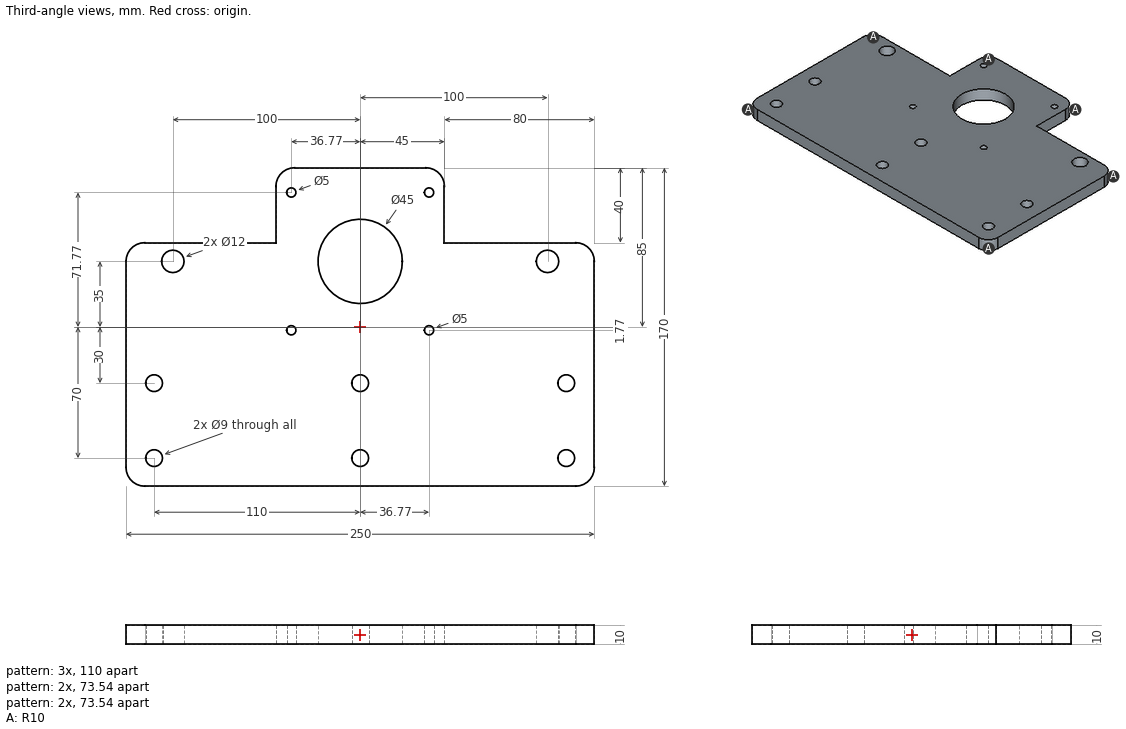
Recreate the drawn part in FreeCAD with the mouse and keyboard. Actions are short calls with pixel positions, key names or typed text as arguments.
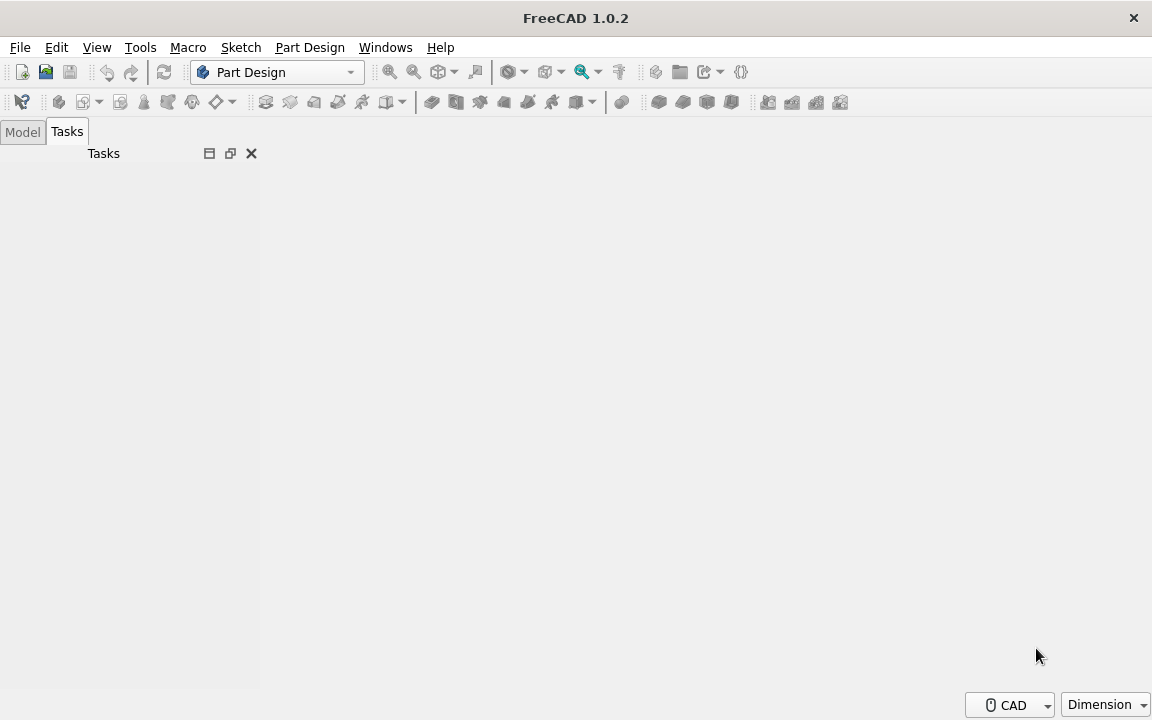
click(22, 72)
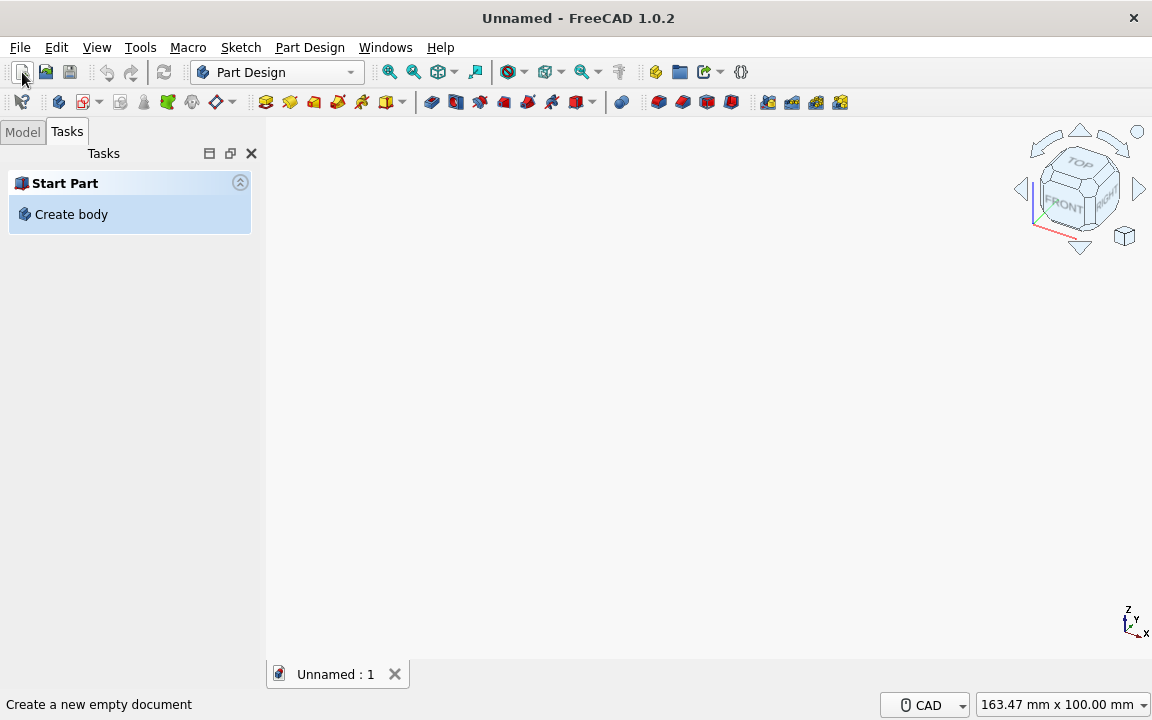
click(84, 102)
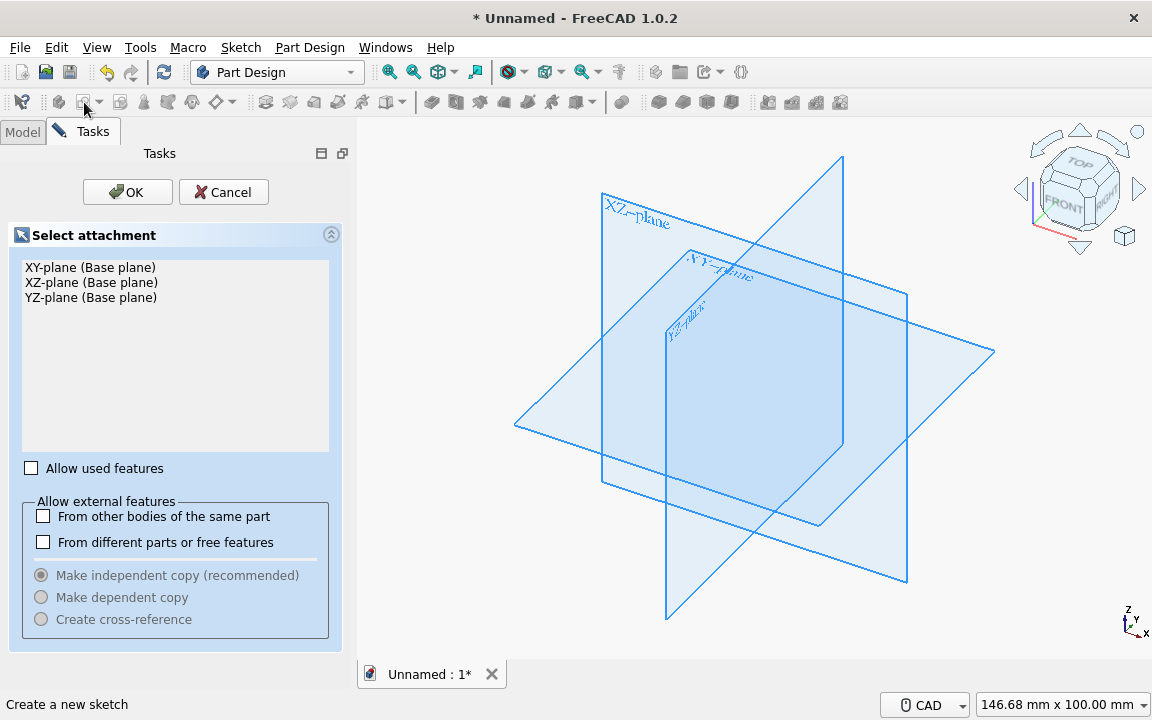
click(82, 268)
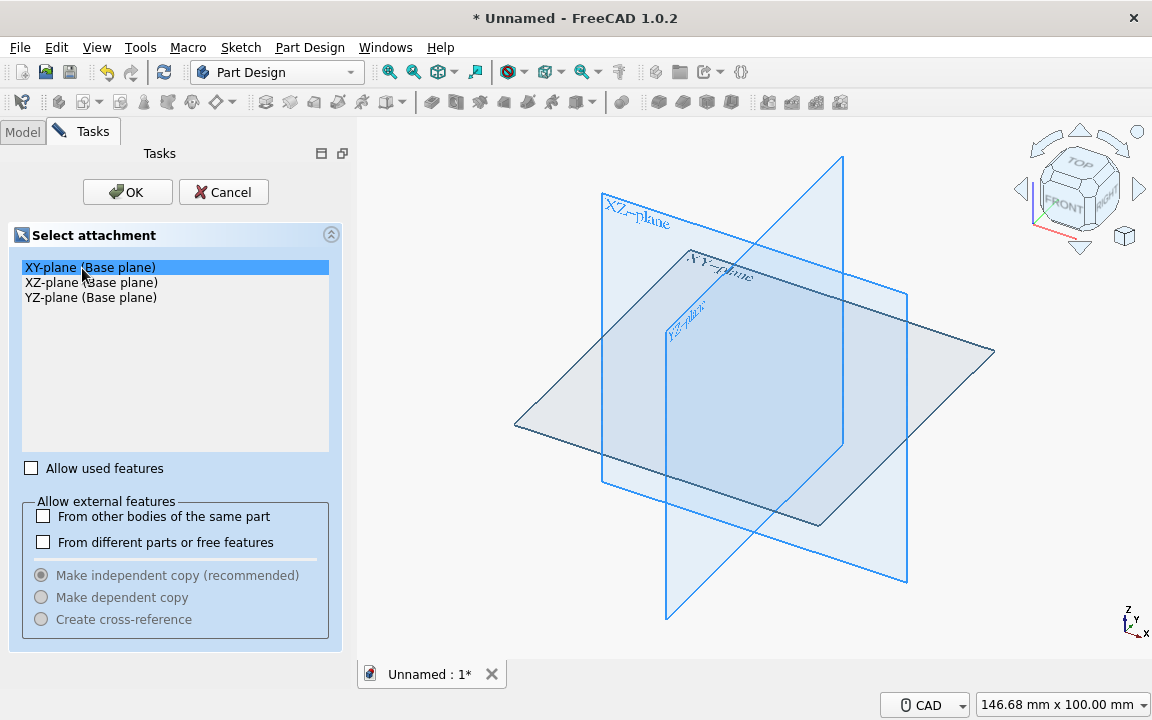
click(128, 192)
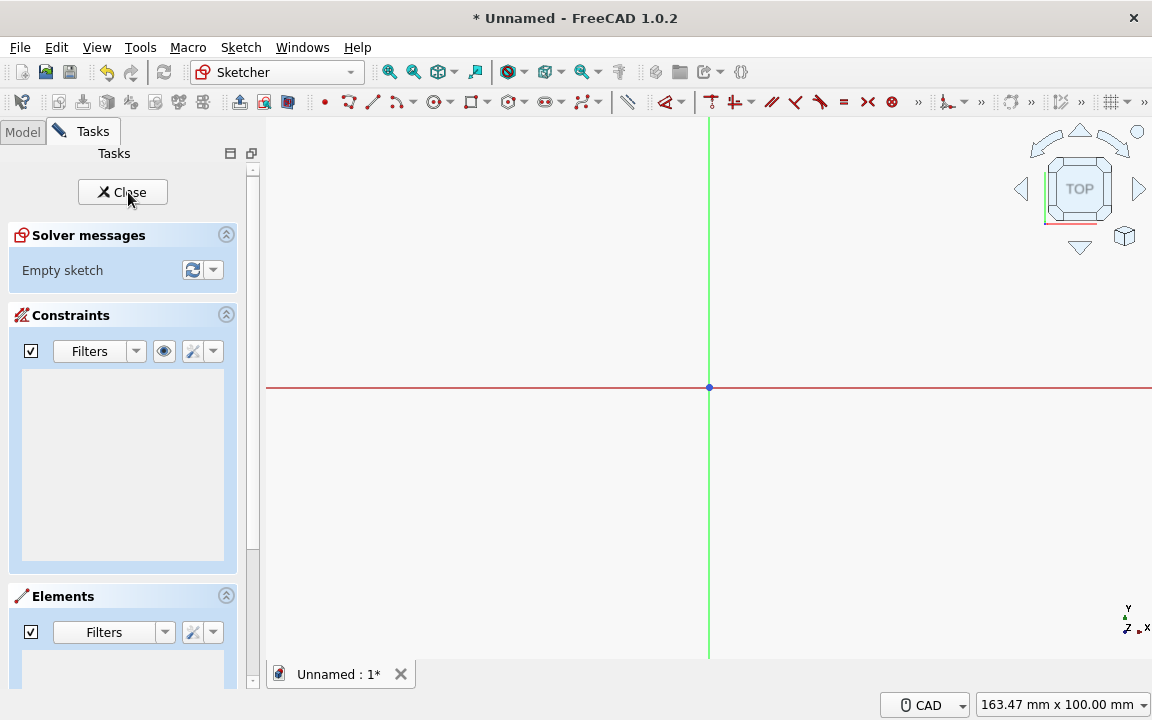
scroll(601, 388, down, 5)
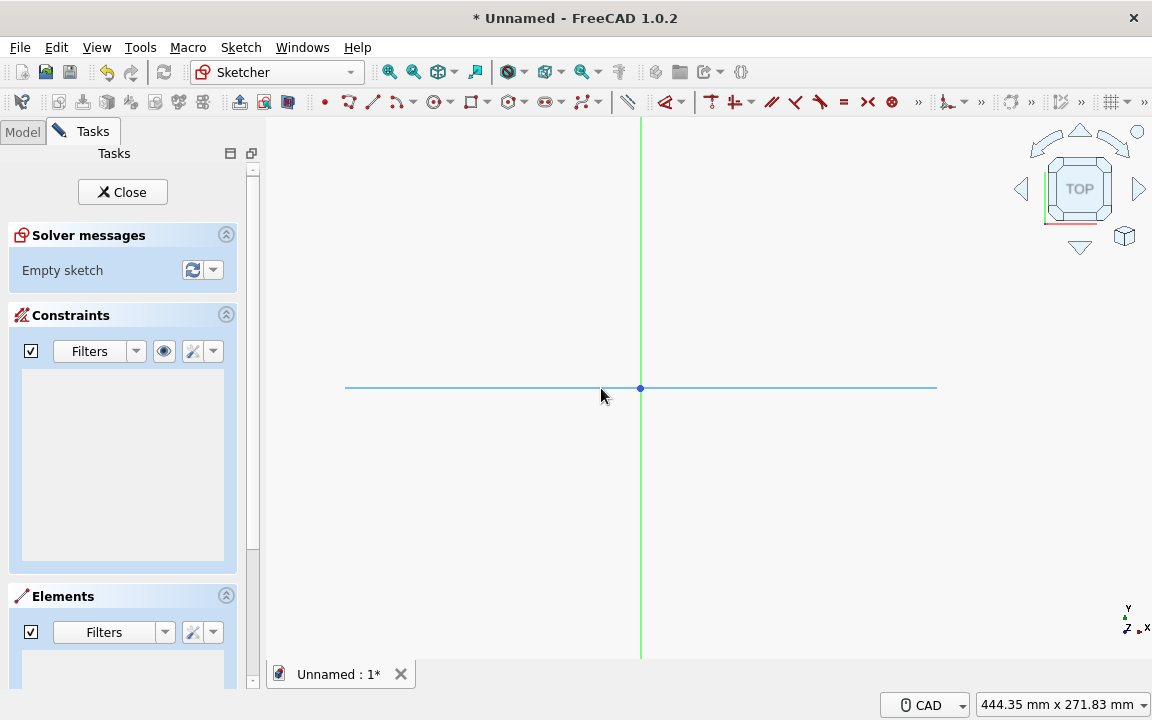
key(g)
key(v)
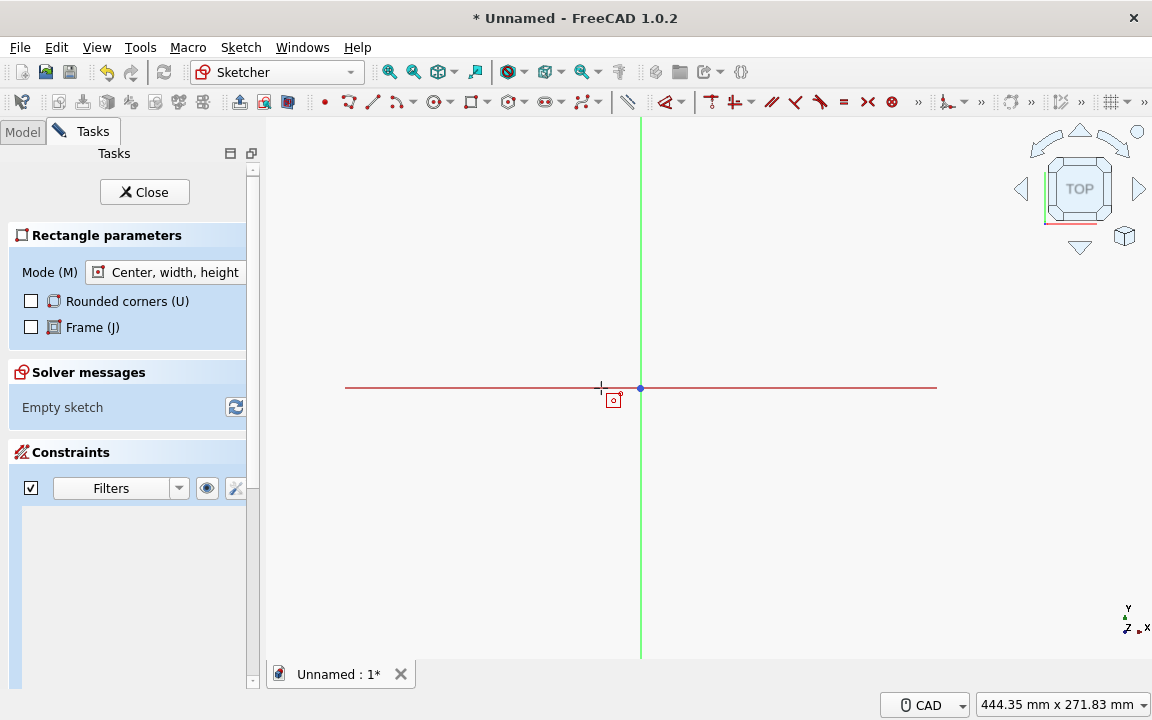
click(641, 388)
move(890, 219)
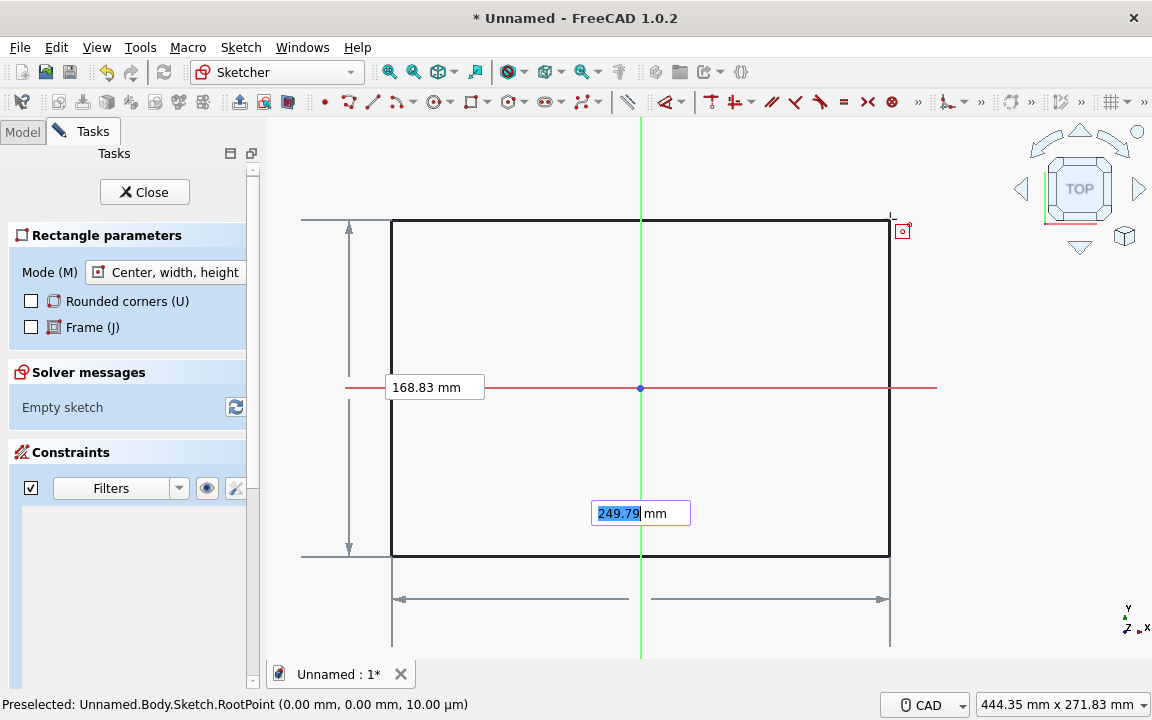
text(250)
key(Tab)
text(170)
key(Return)
key(Escape)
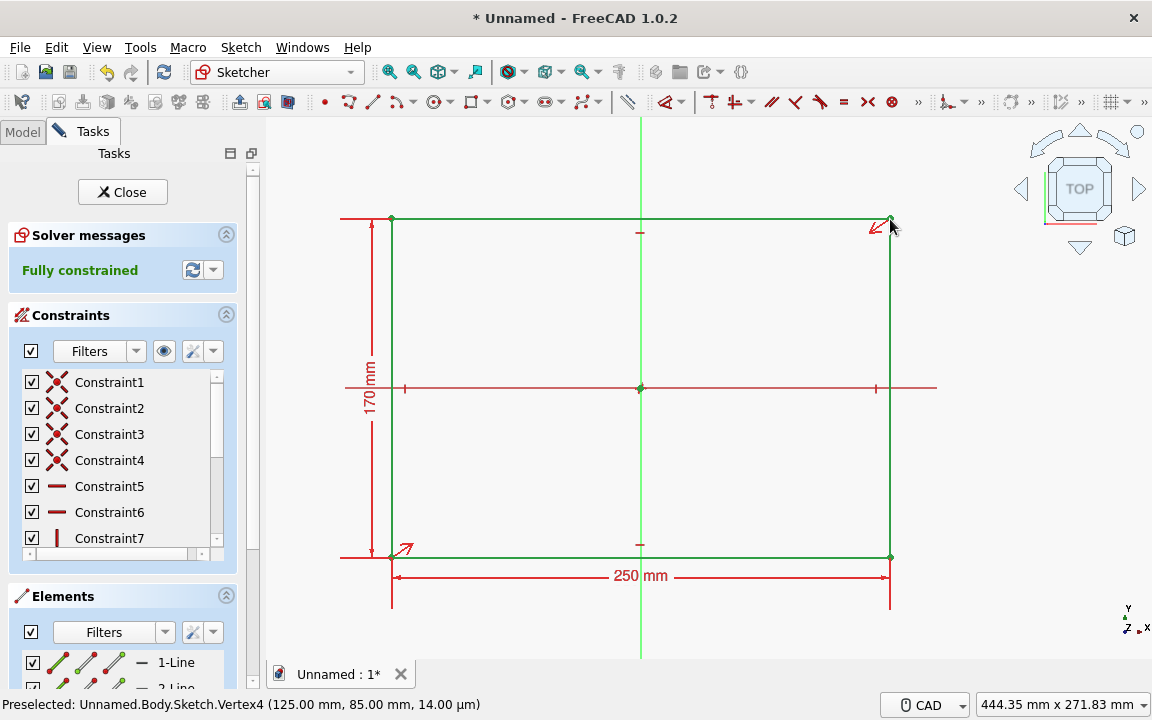
click(123, 192)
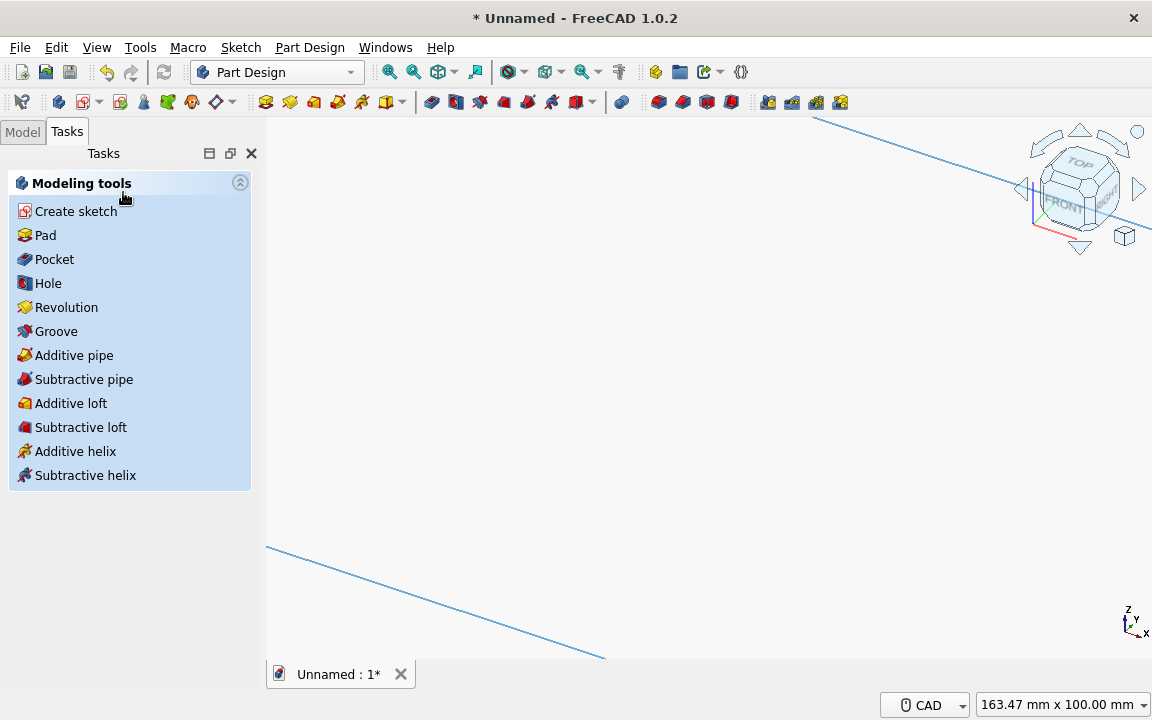
click(266, 102)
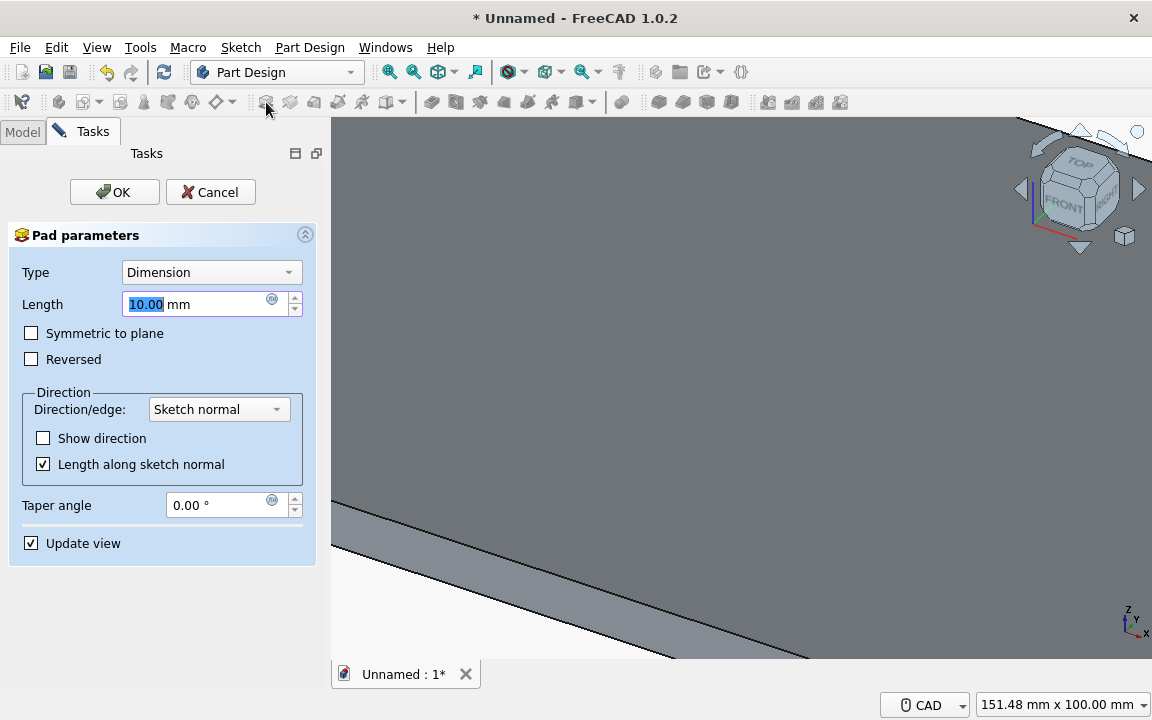
text(10)
key(Tab)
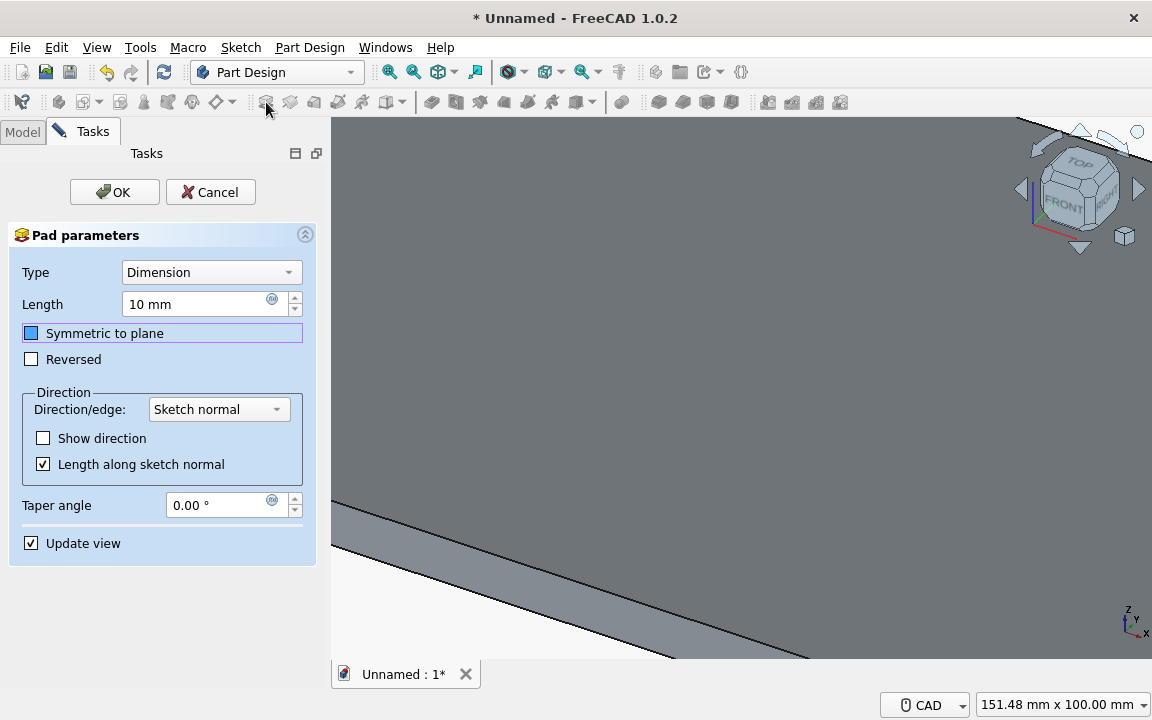
click(30, 333)